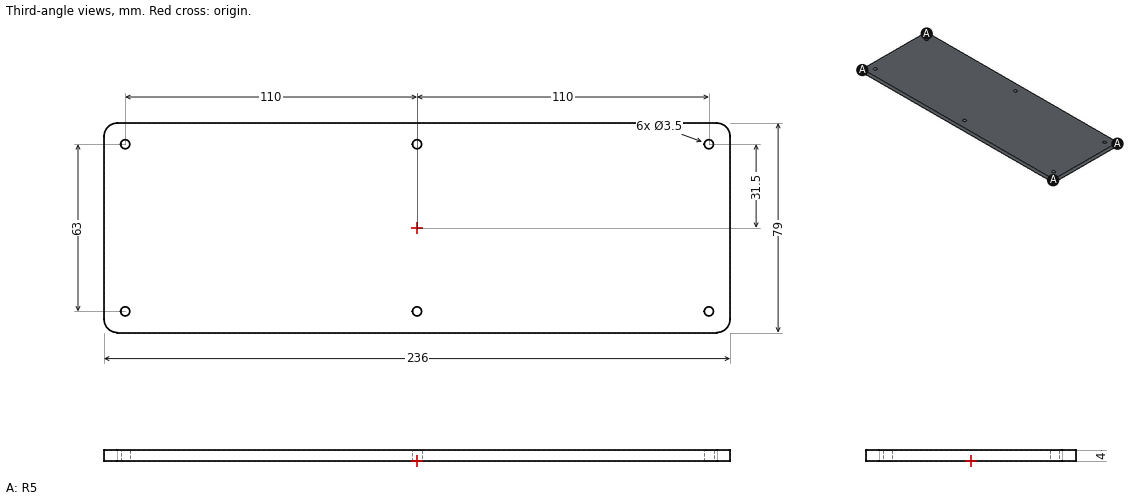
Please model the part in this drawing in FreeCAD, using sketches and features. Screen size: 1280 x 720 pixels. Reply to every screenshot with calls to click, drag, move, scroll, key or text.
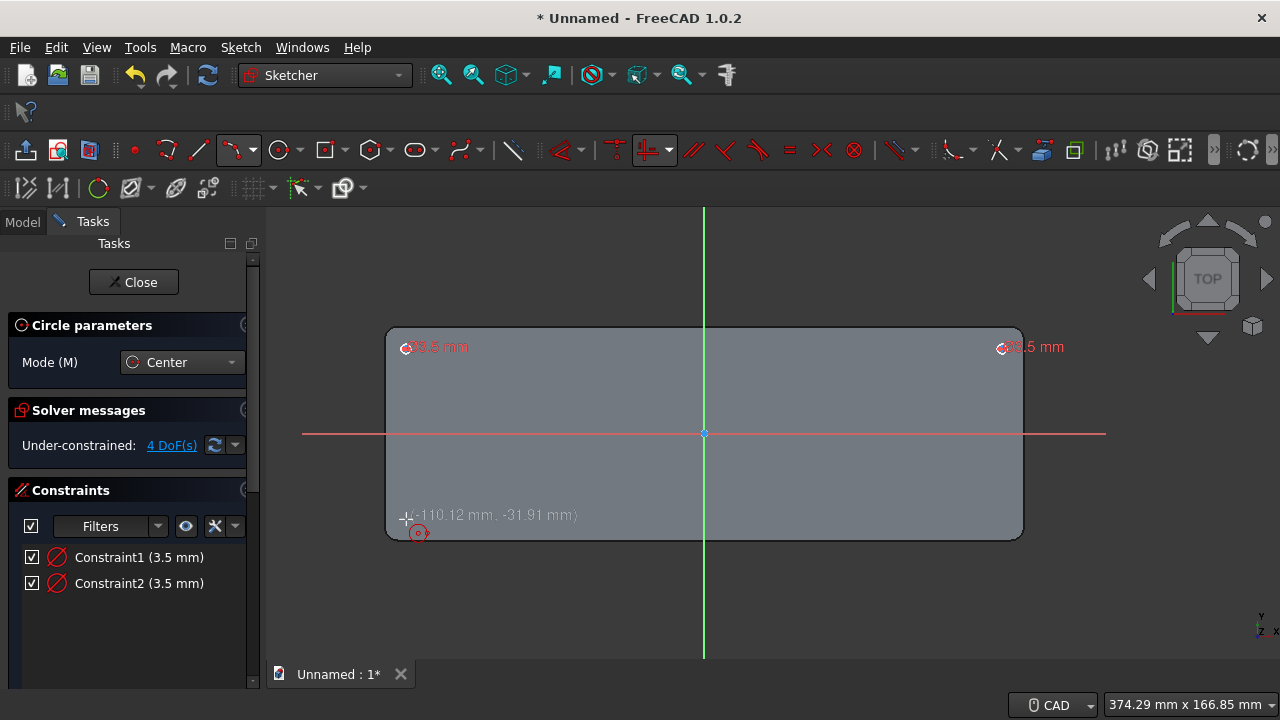
click(406, 519)
move(410, 516)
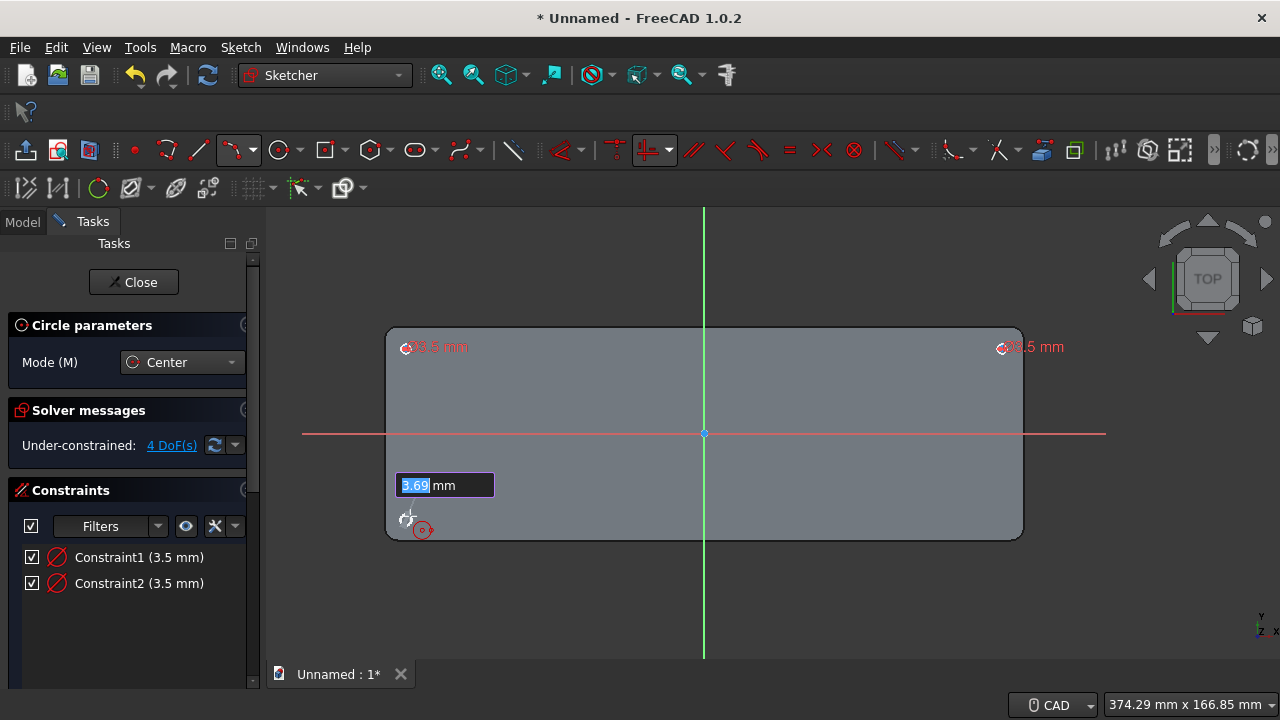
text(3.5)
key(Return)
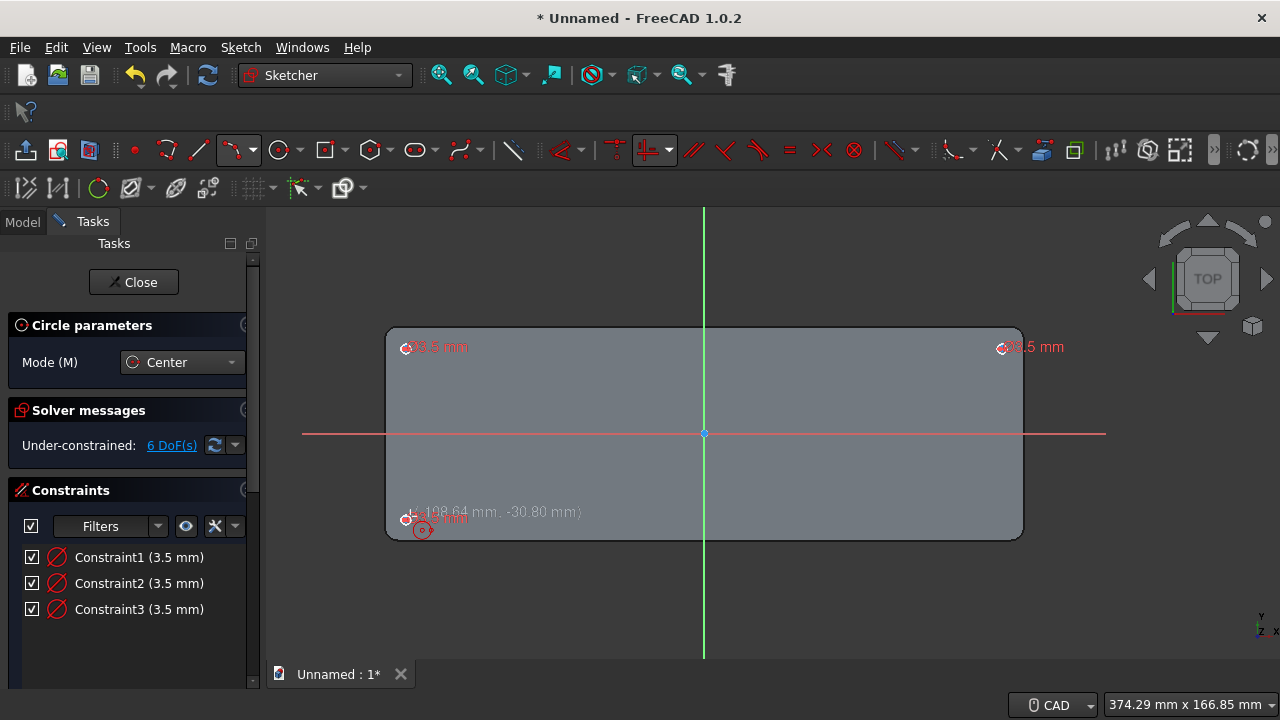
scroll(1002, 519, up, 8)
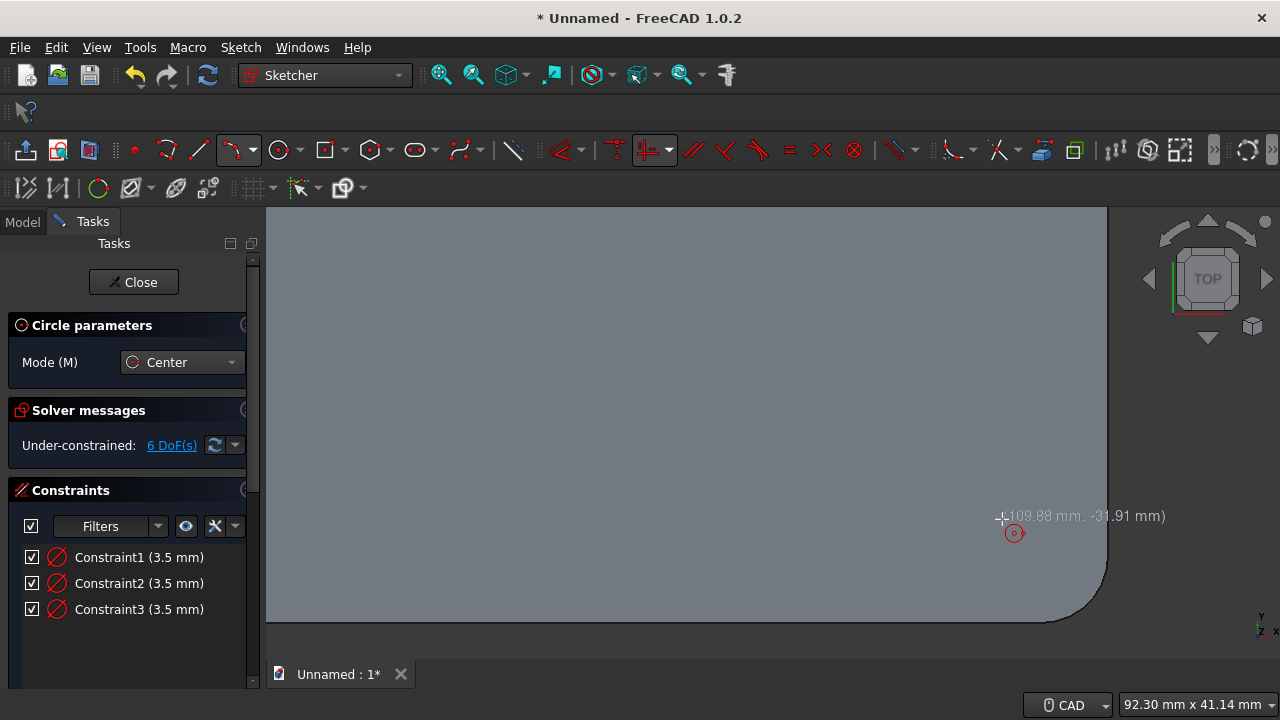
scroll(1003, 519, down, 8)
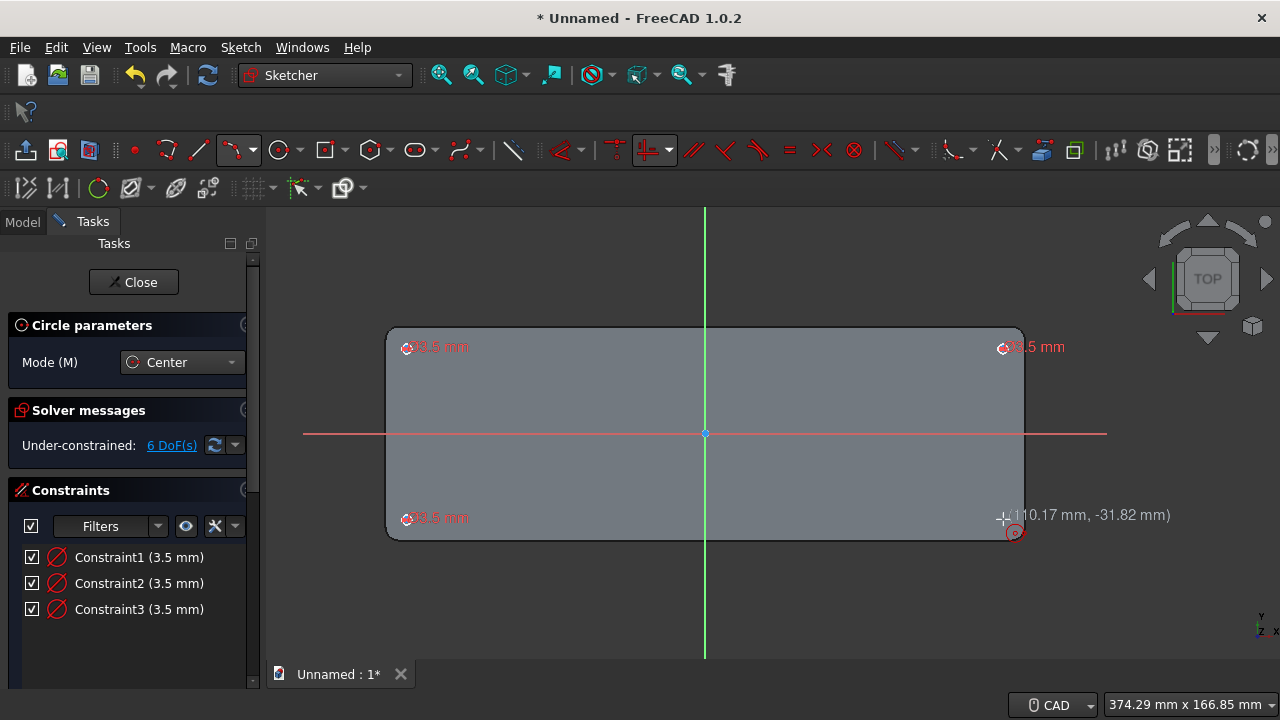
click(1003, 519)
move(1006, 516)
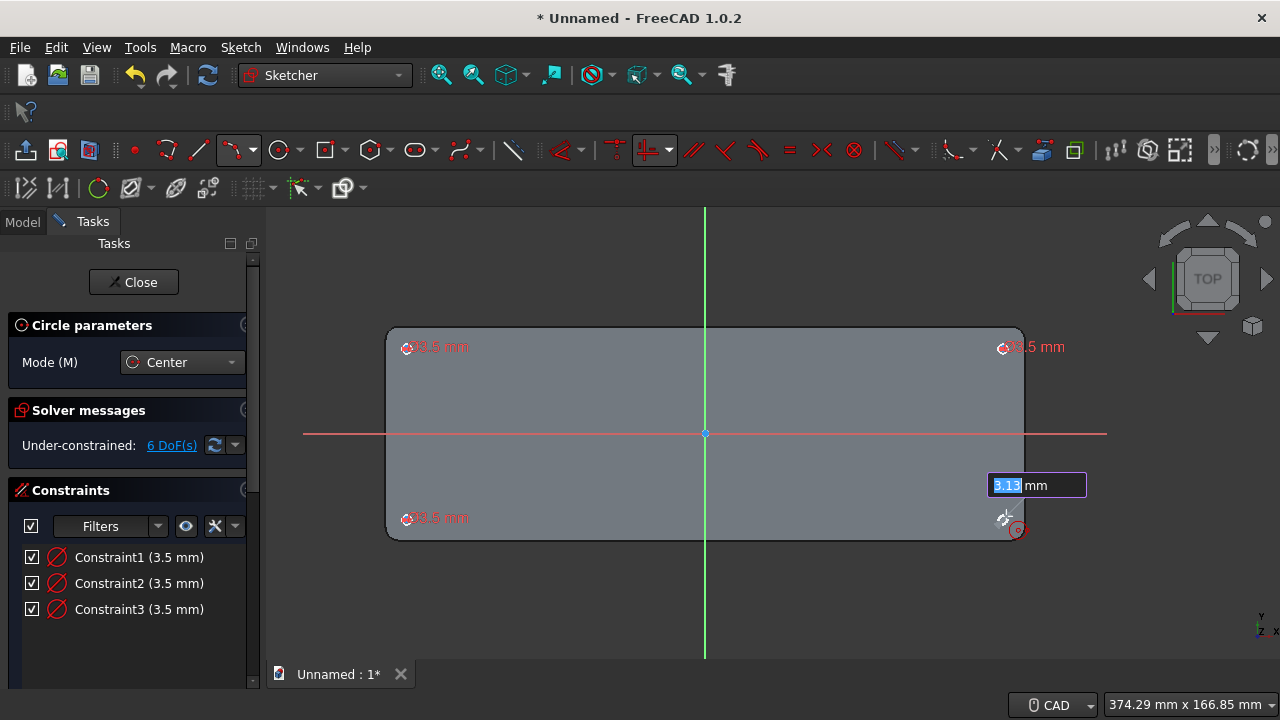
text(3.5)
key(Return)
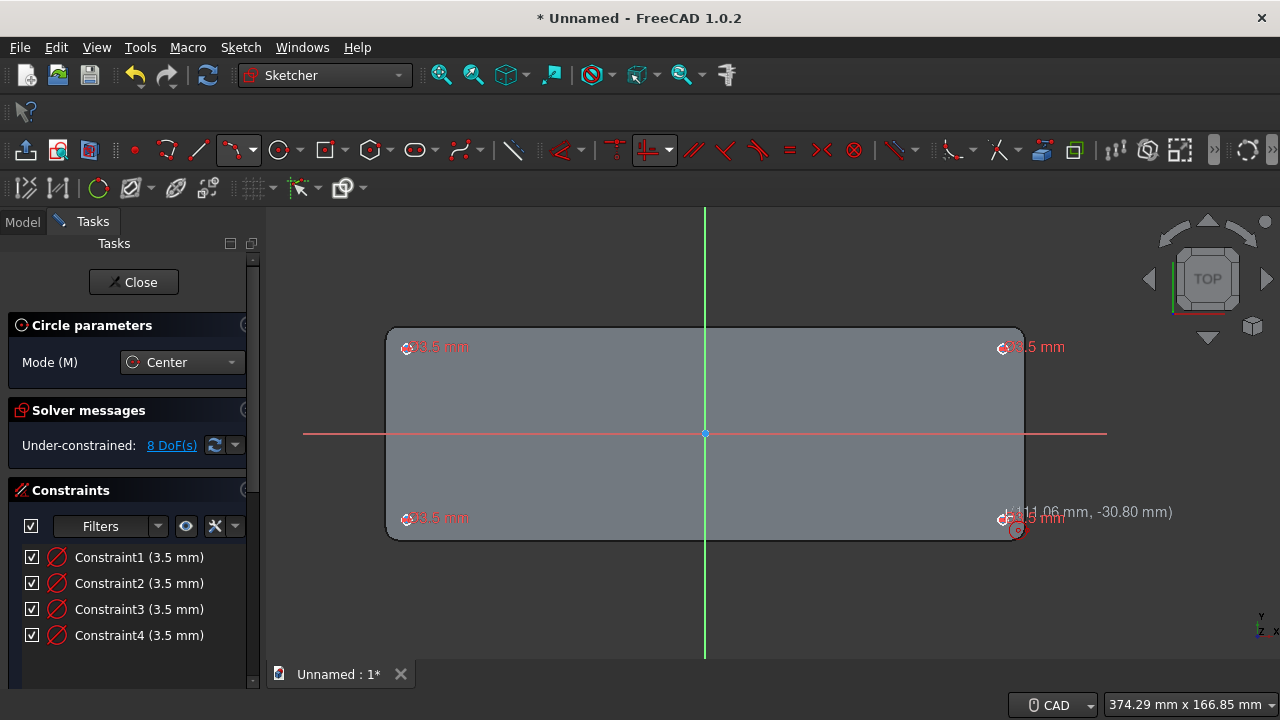
scroll(705, 348, up, 8)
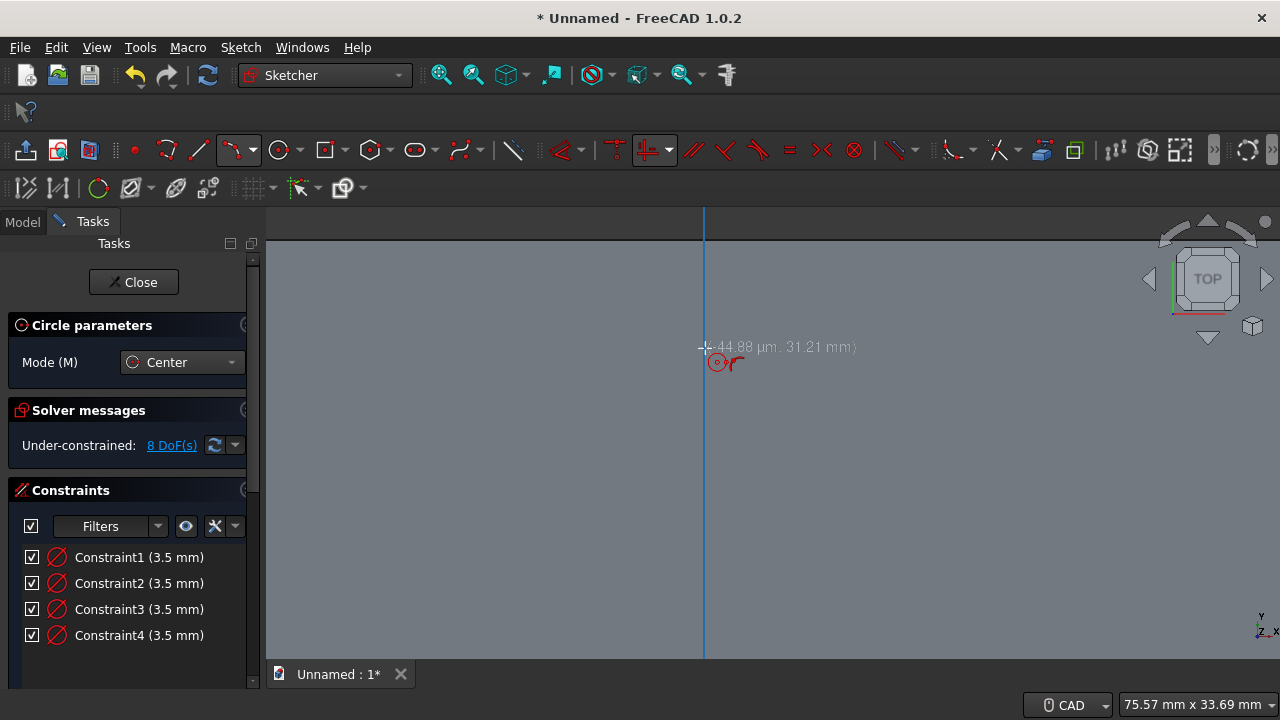
scroll(705, 348, down, 8)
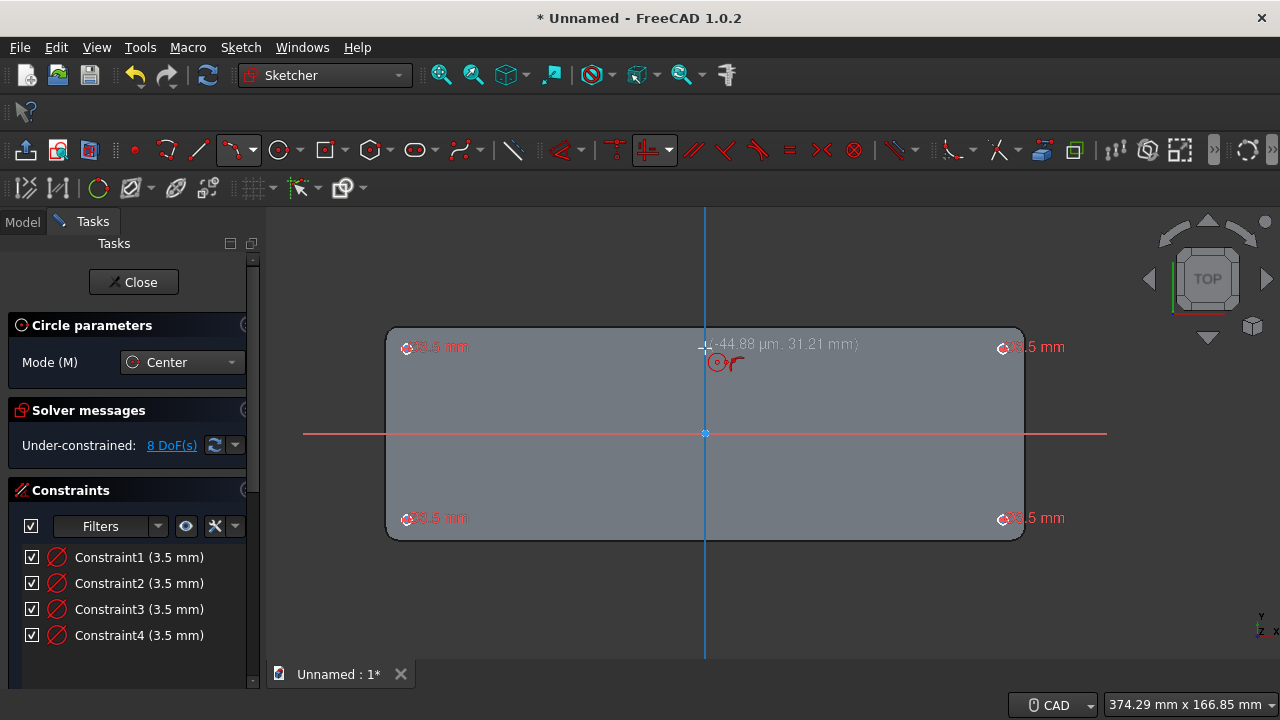
click(705, 348)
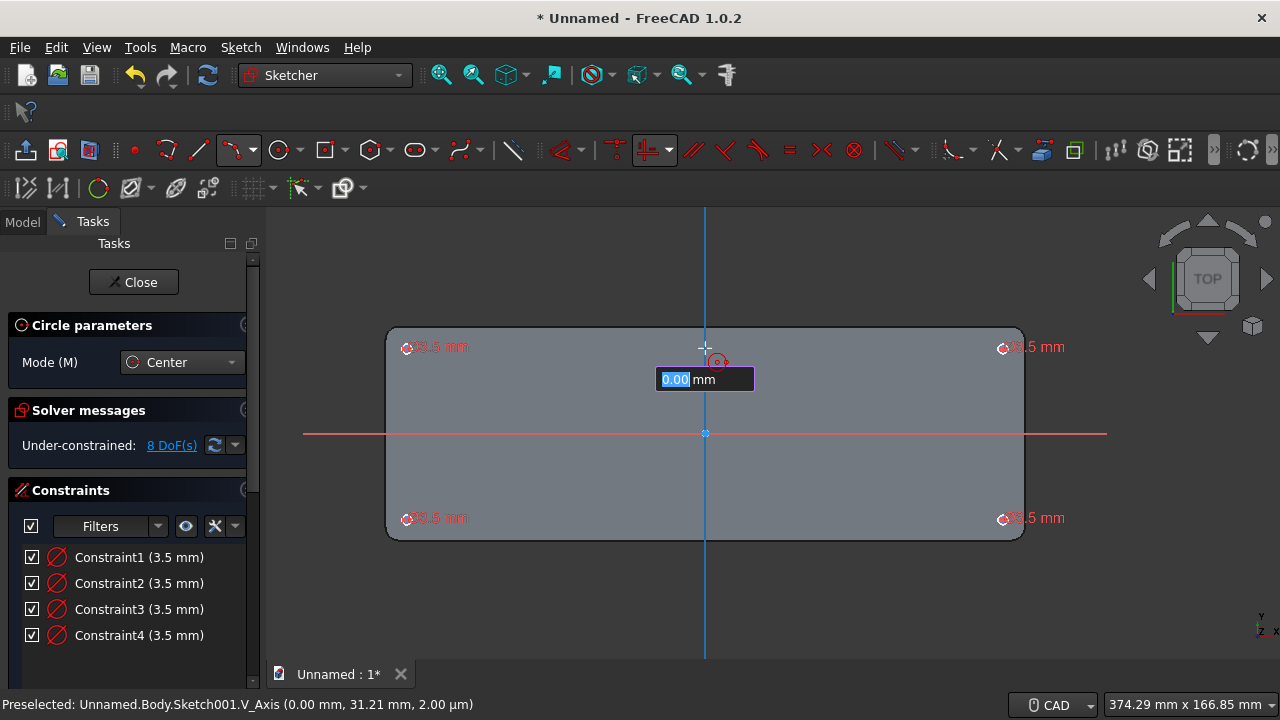
scroll(710, 347, up, 7)
move(707, 344)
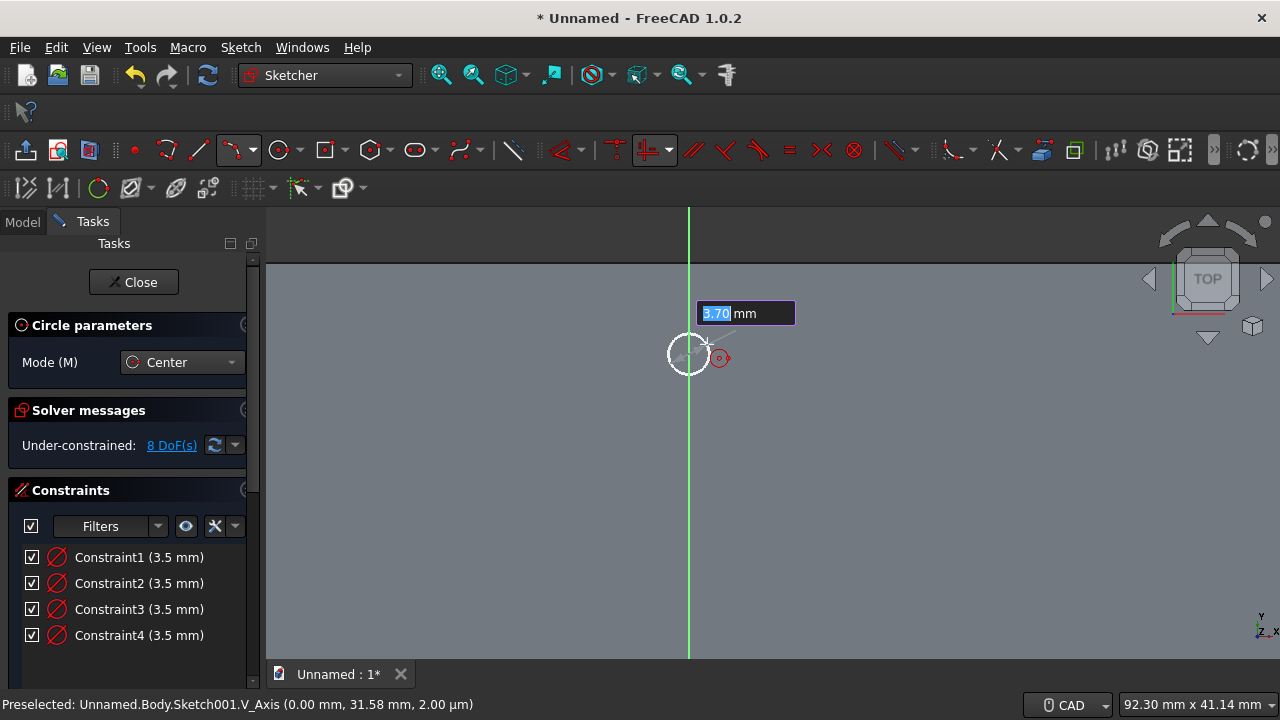
text(3.5)
key(Return)